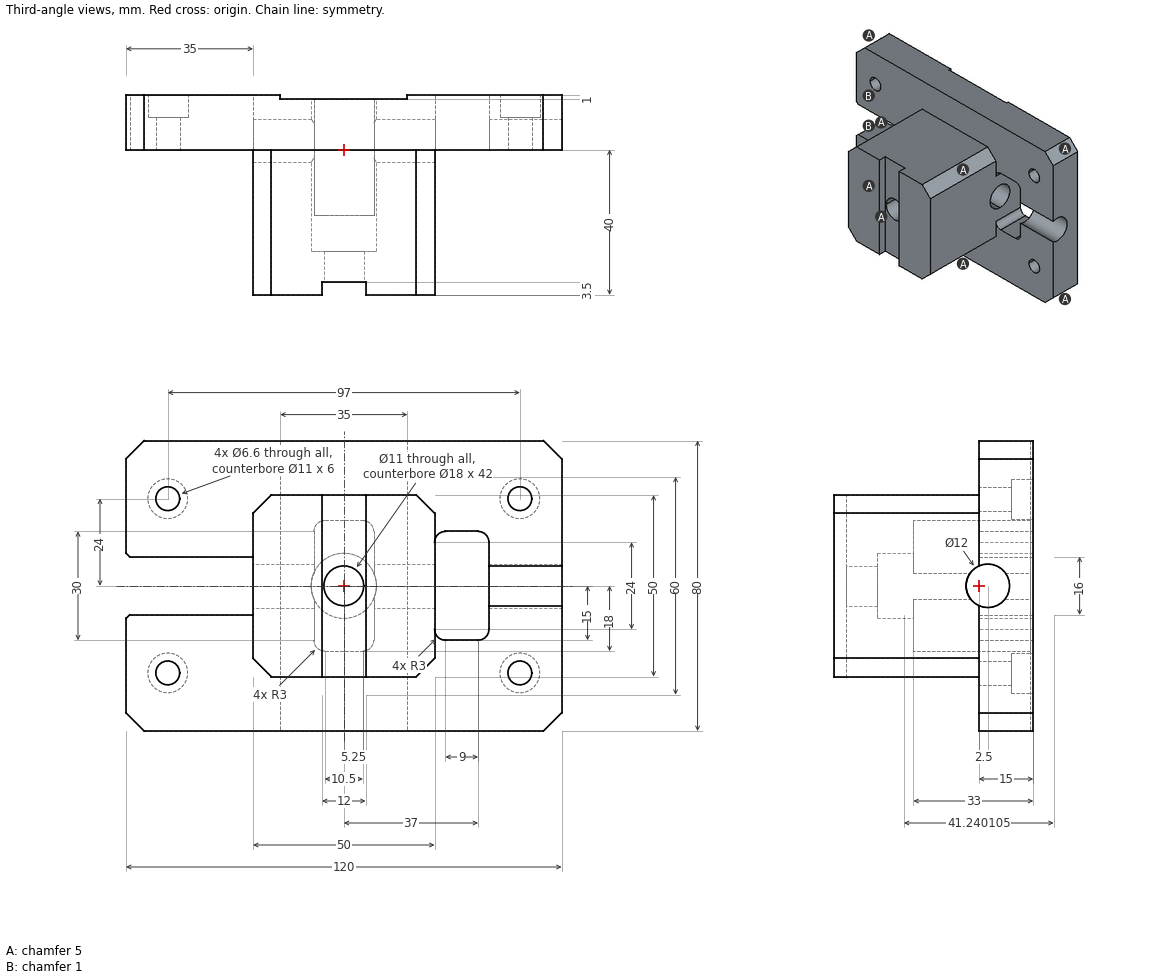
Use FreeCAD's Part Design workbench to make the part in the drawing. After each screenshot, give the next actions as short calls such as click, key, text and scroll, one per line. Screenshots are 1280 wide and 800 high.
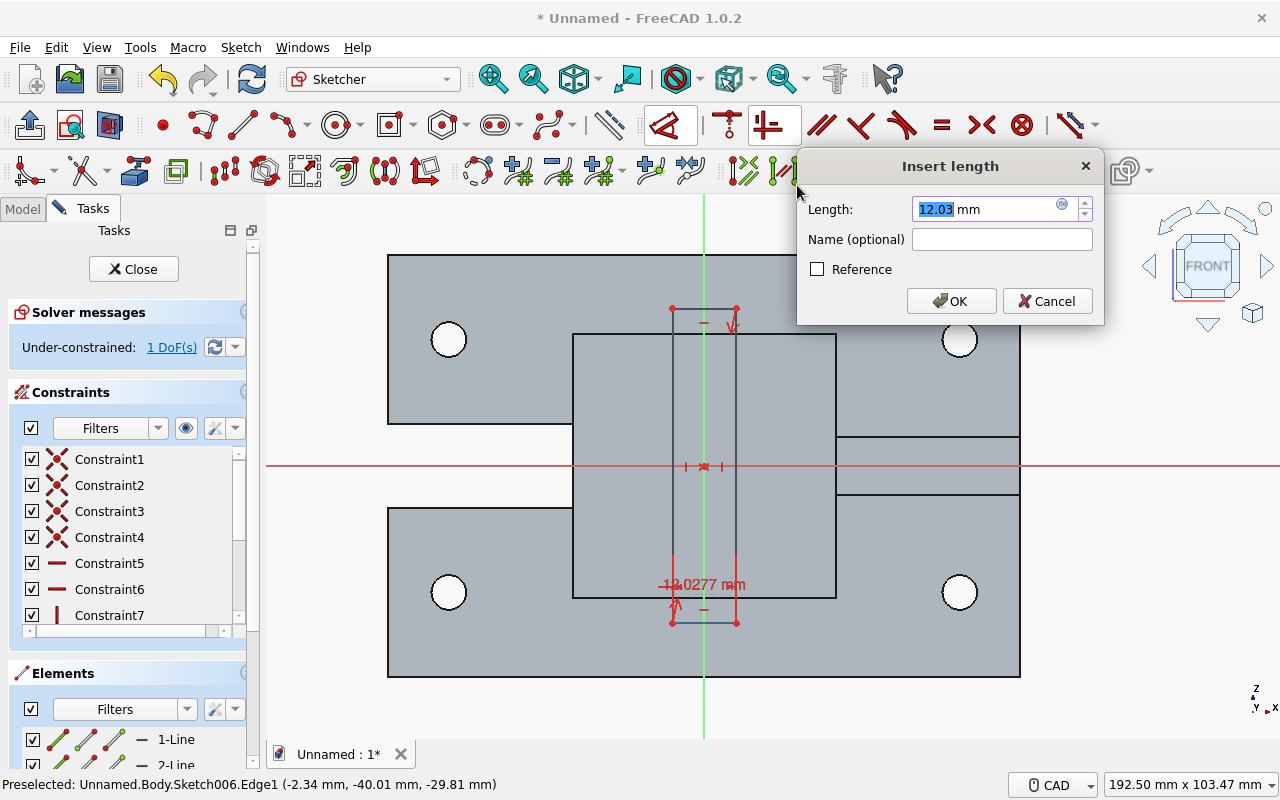
text(12)
key(Return)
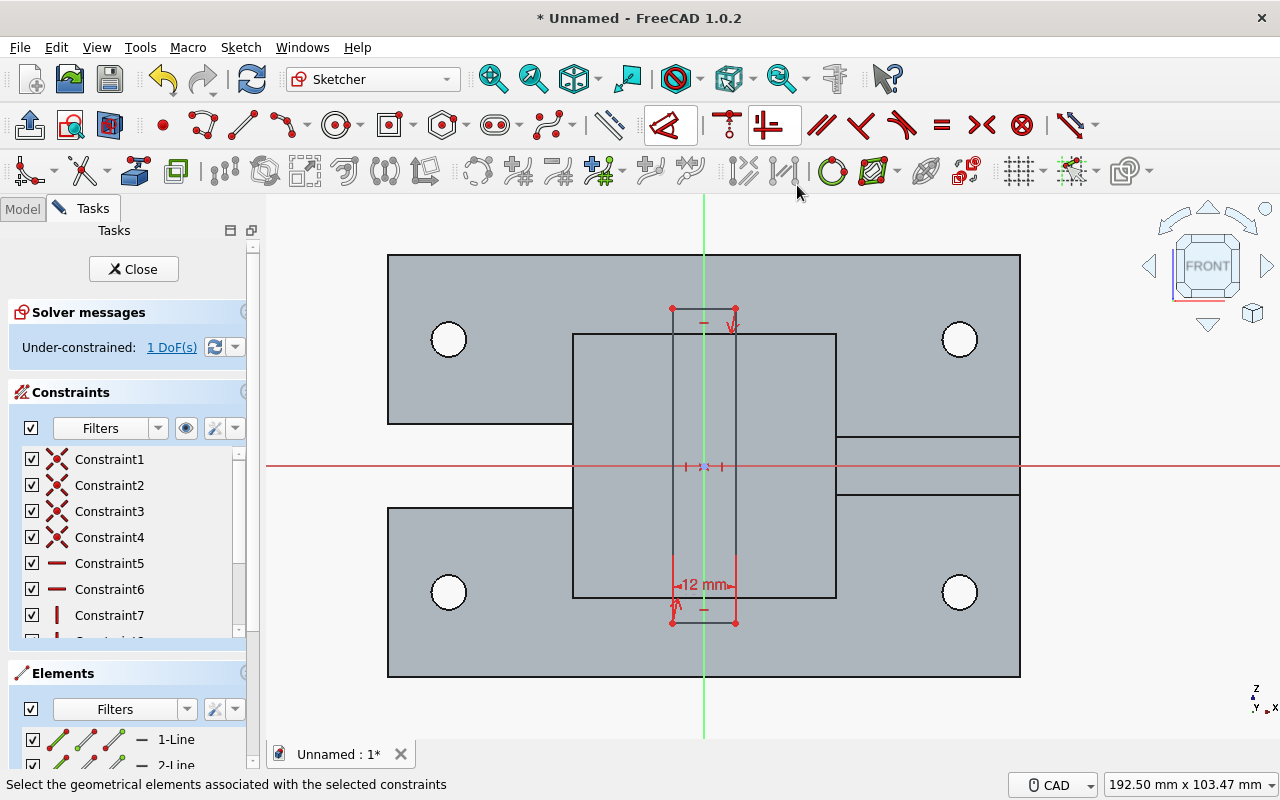
click(736, 529)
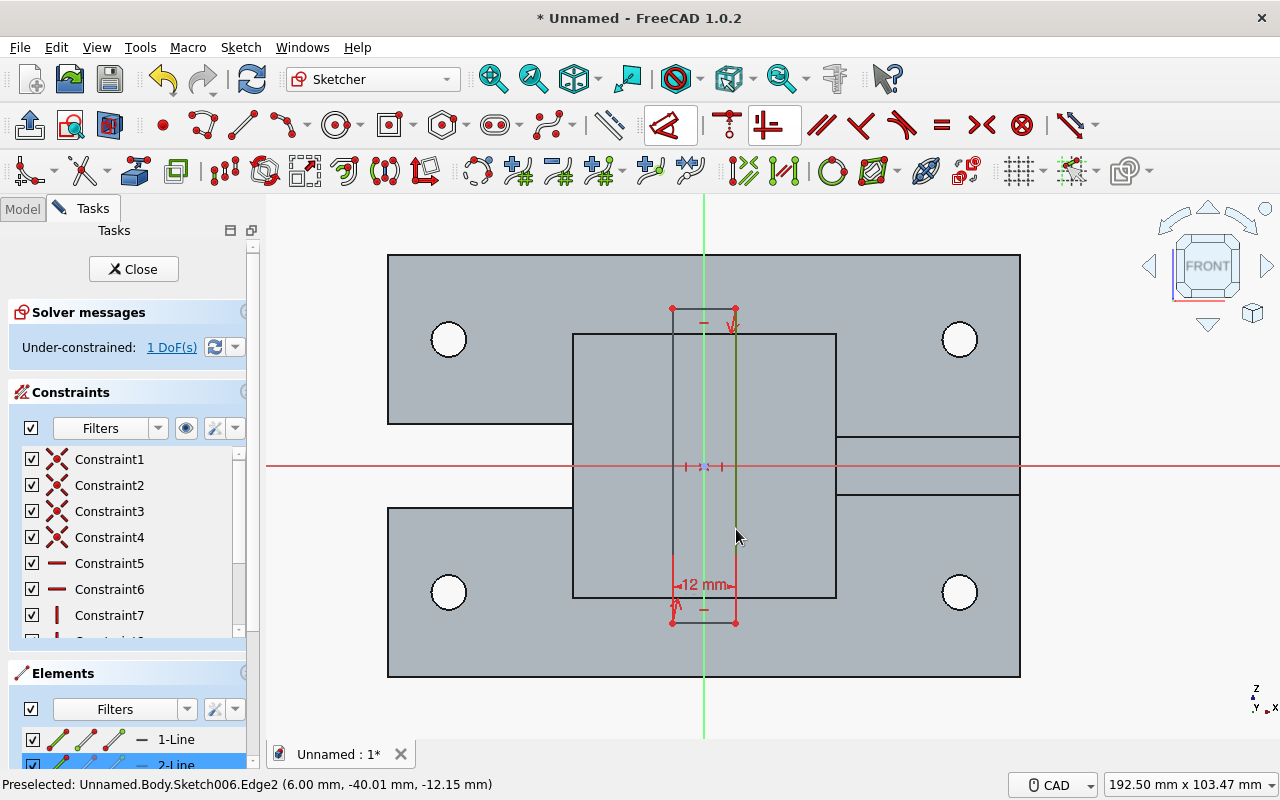
key(i)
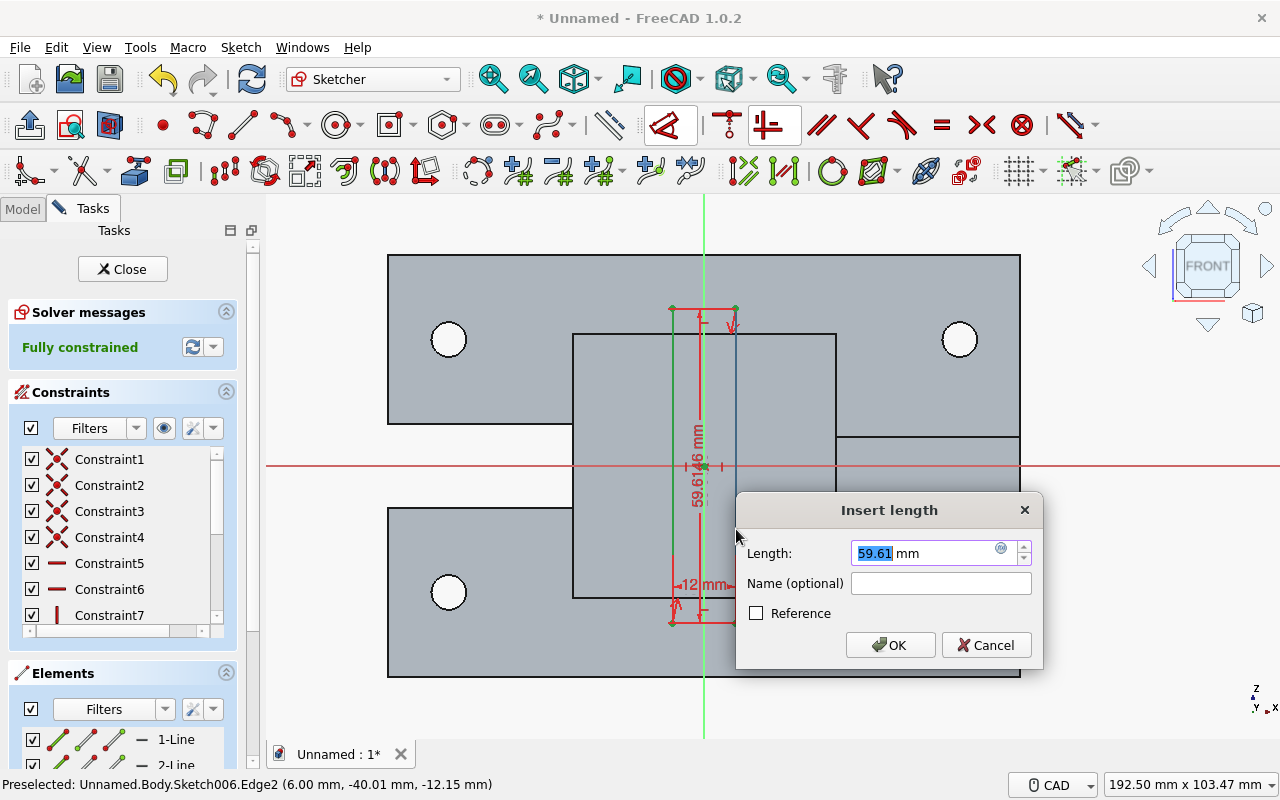
text(60)
key(Return)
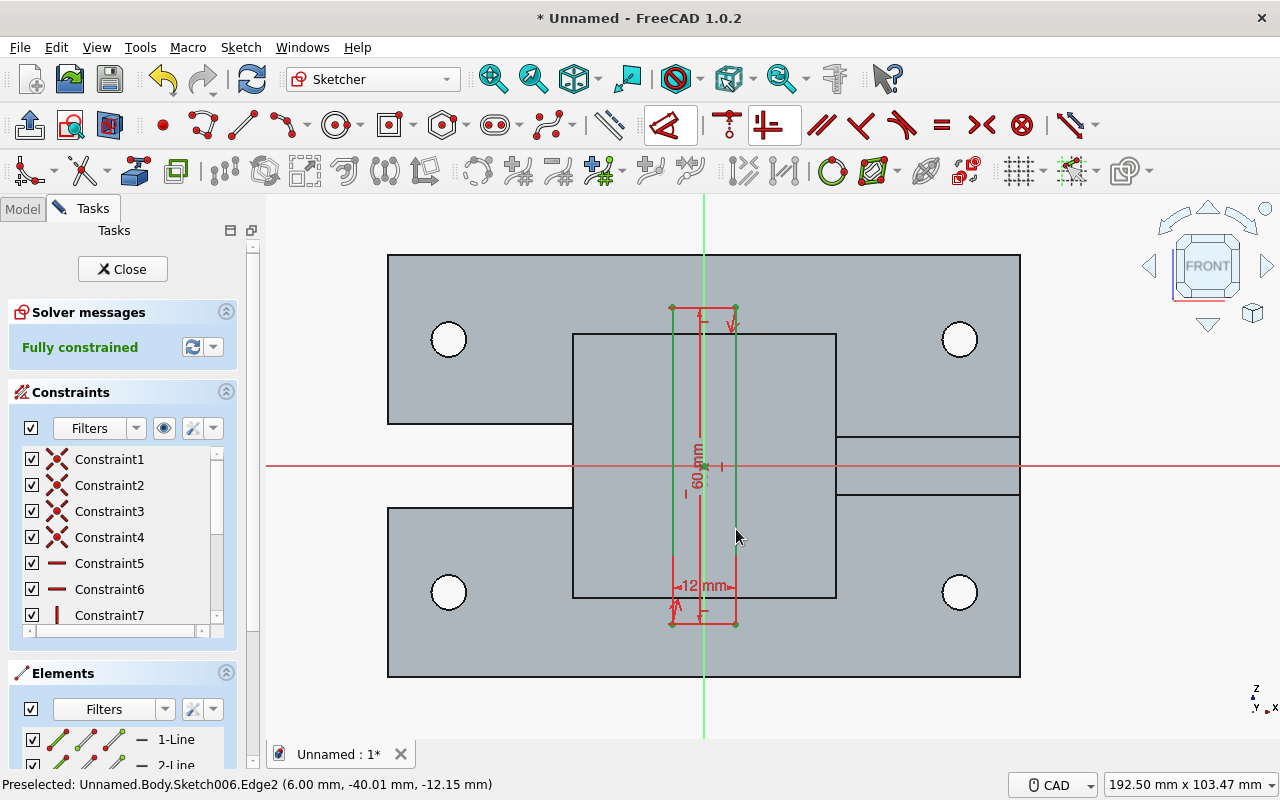
click(123, 269)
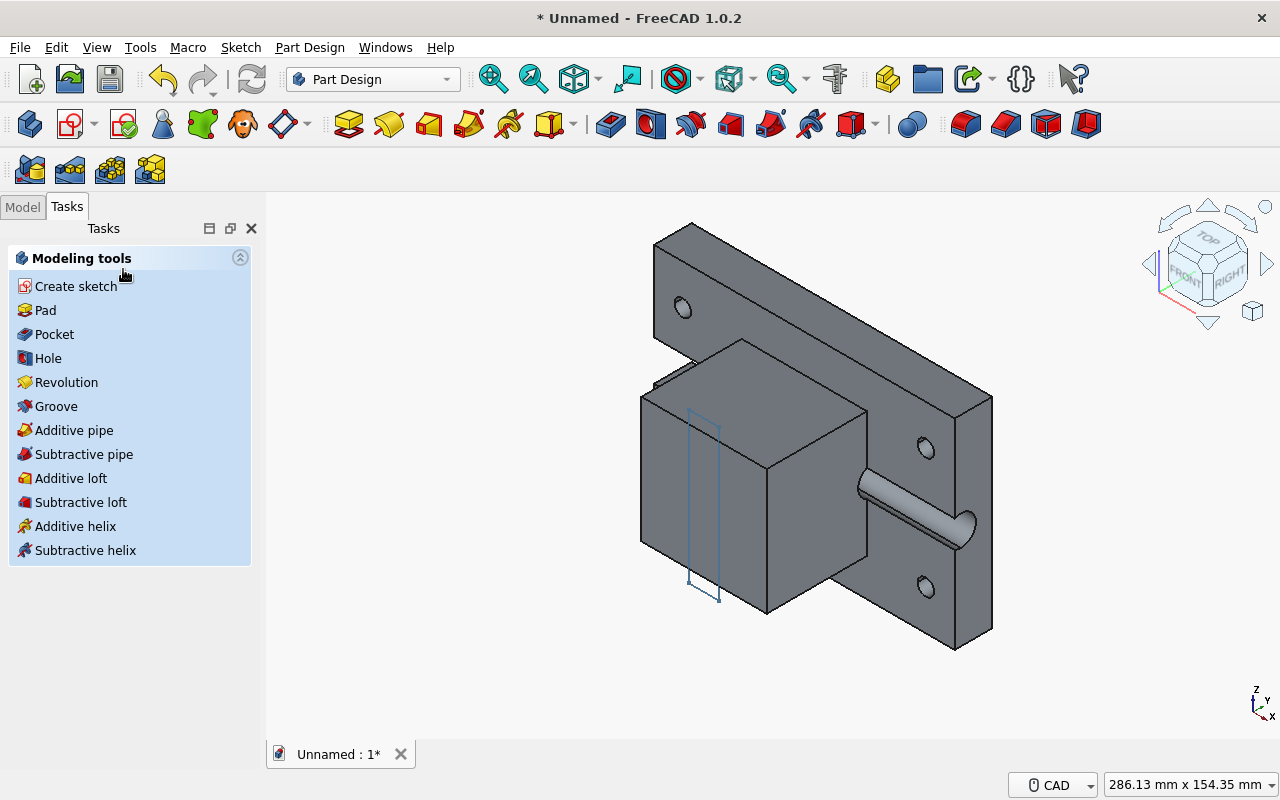
click(612, 124)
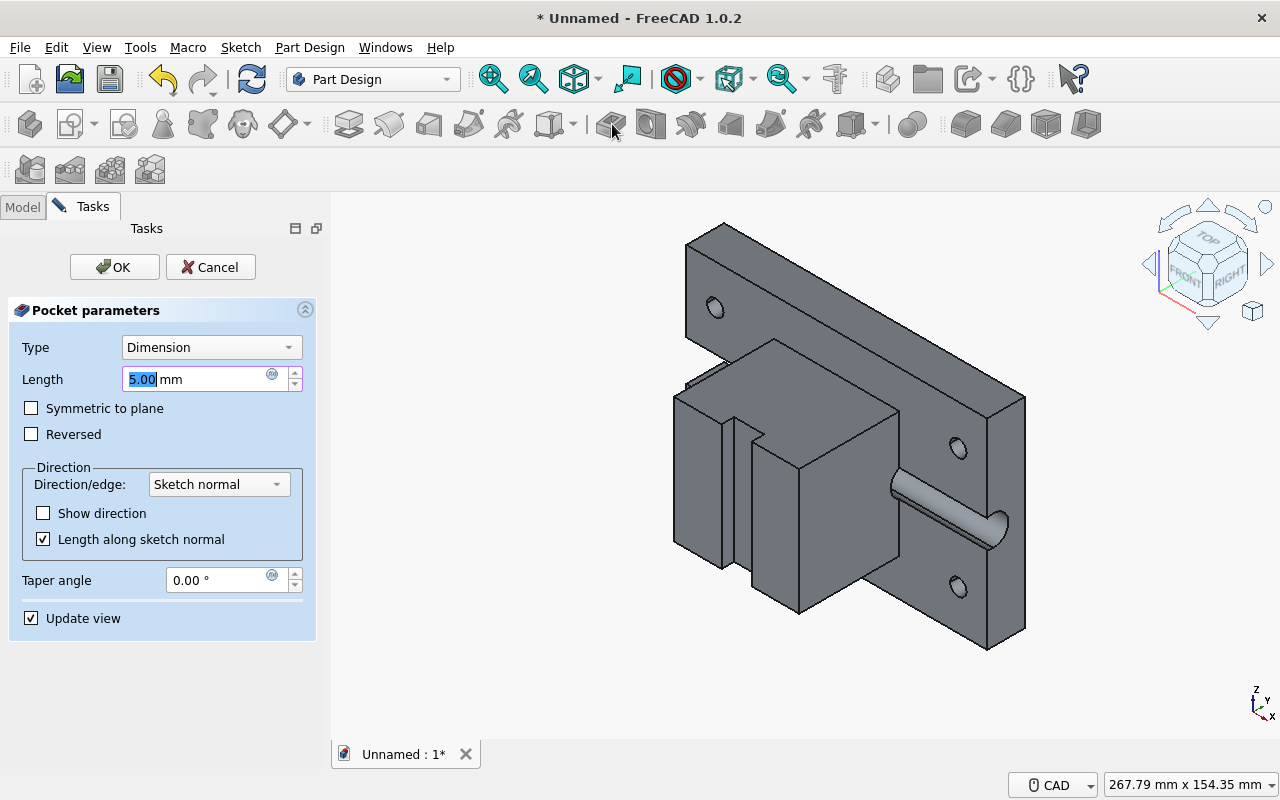
text(3.5)
key(Tab)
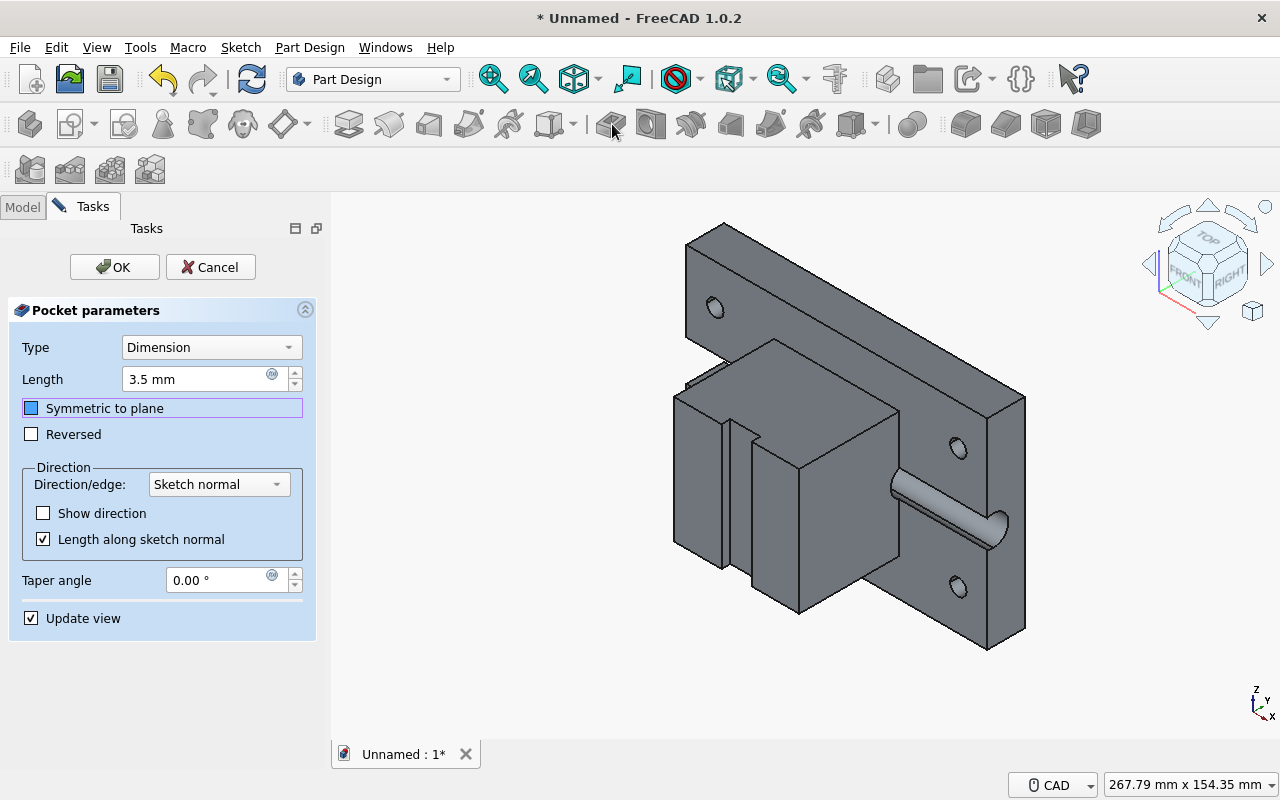
click(115, 267)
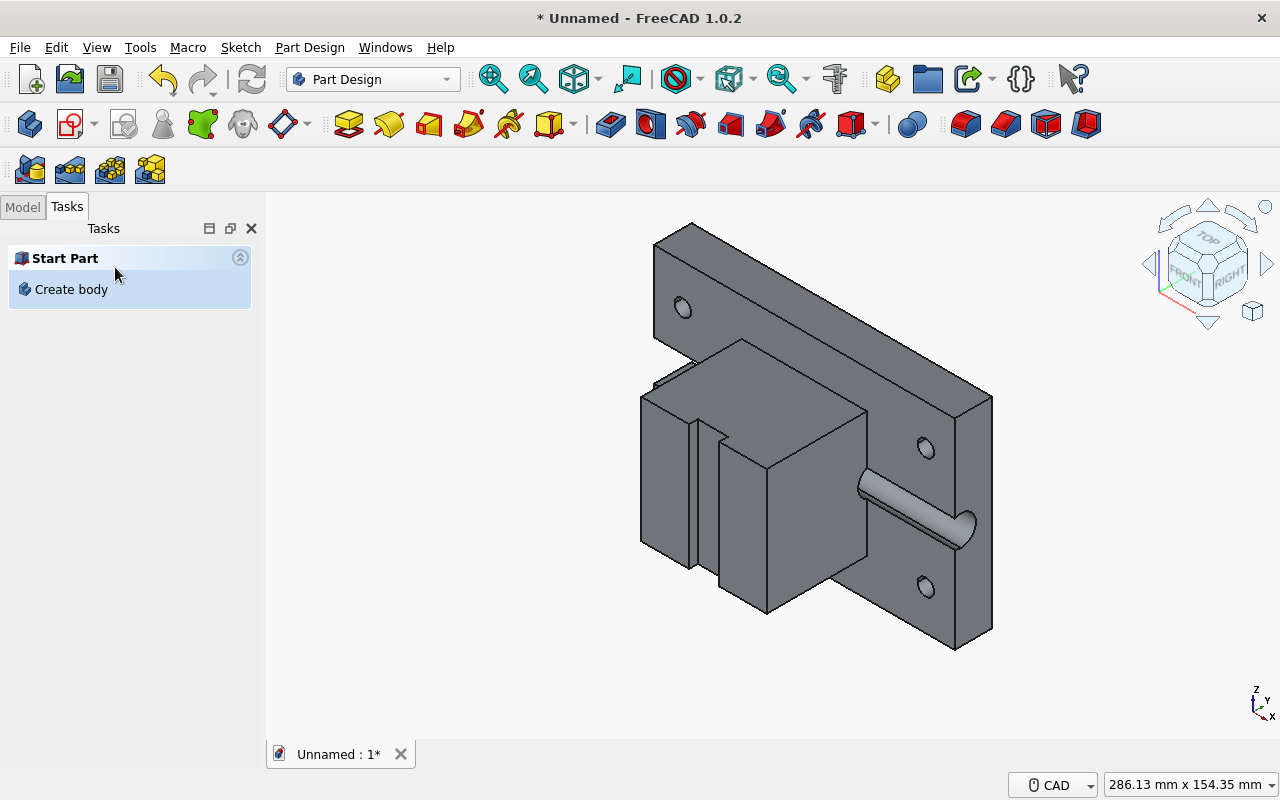
key(4)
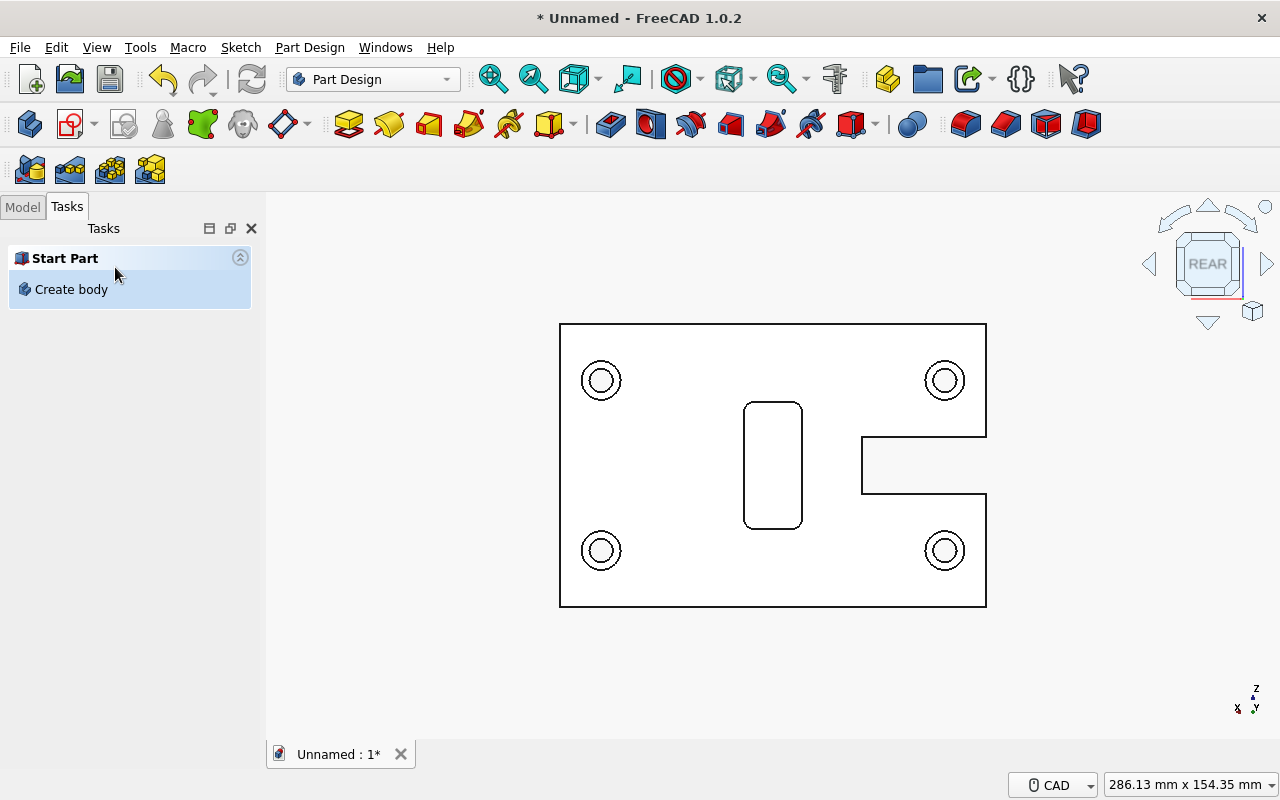
click(651, 465)